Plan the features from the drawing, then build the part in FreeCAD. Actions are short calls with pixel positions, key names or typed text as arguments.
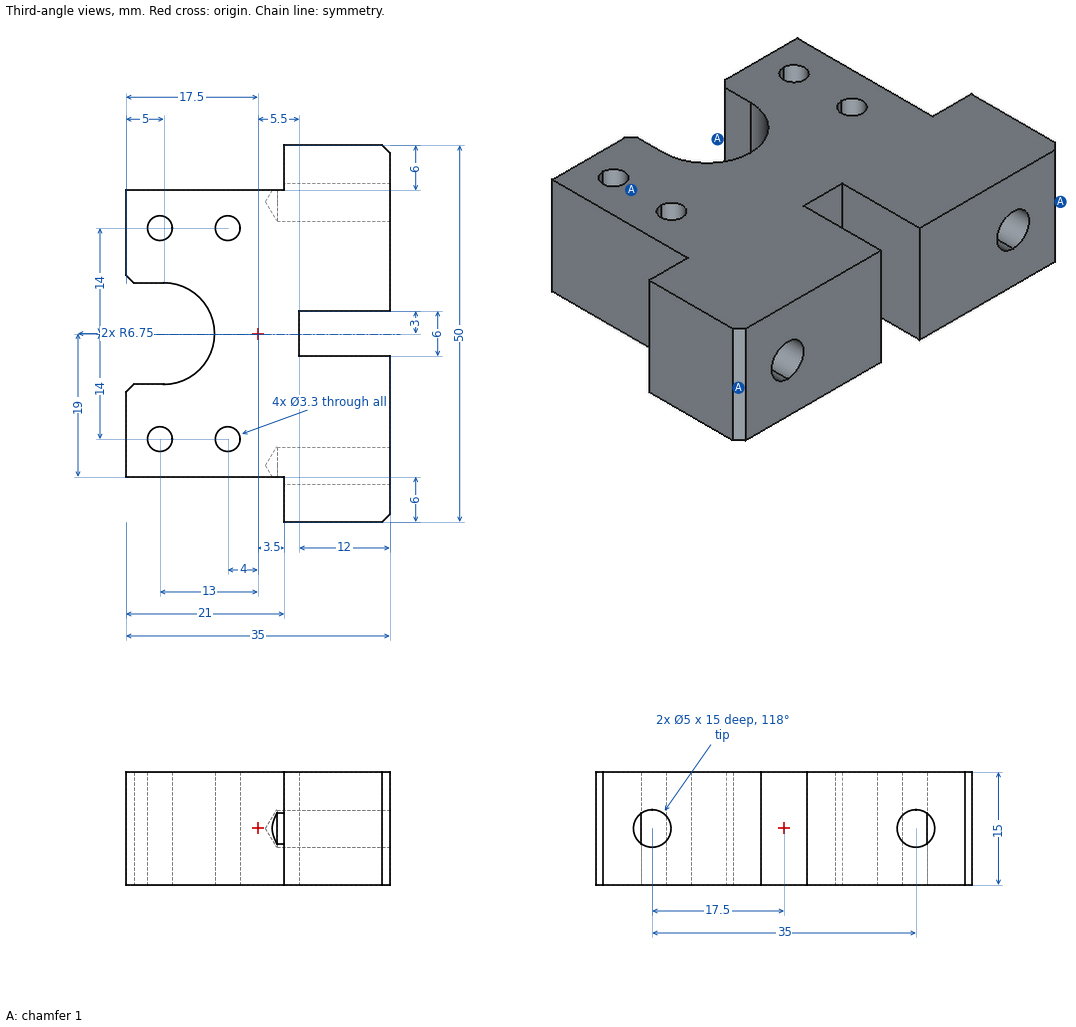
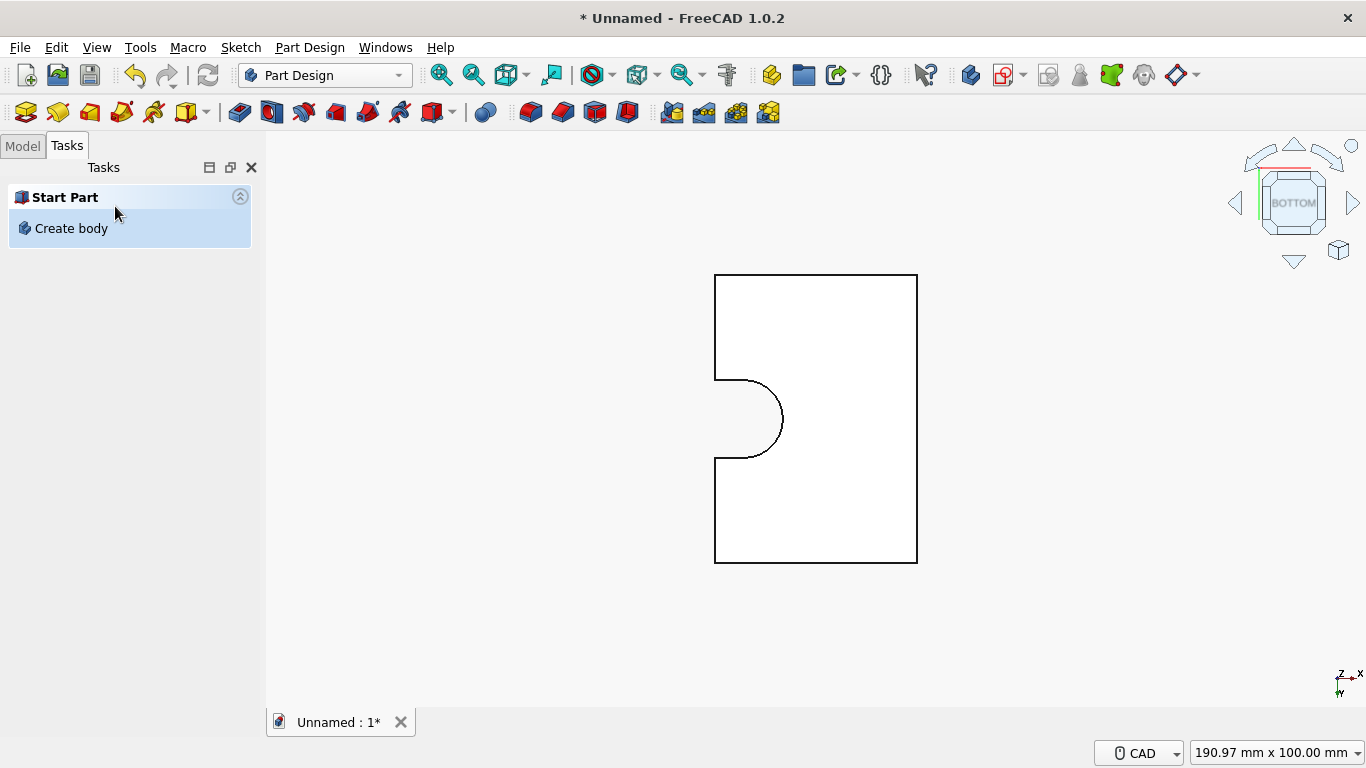
click(845, 459)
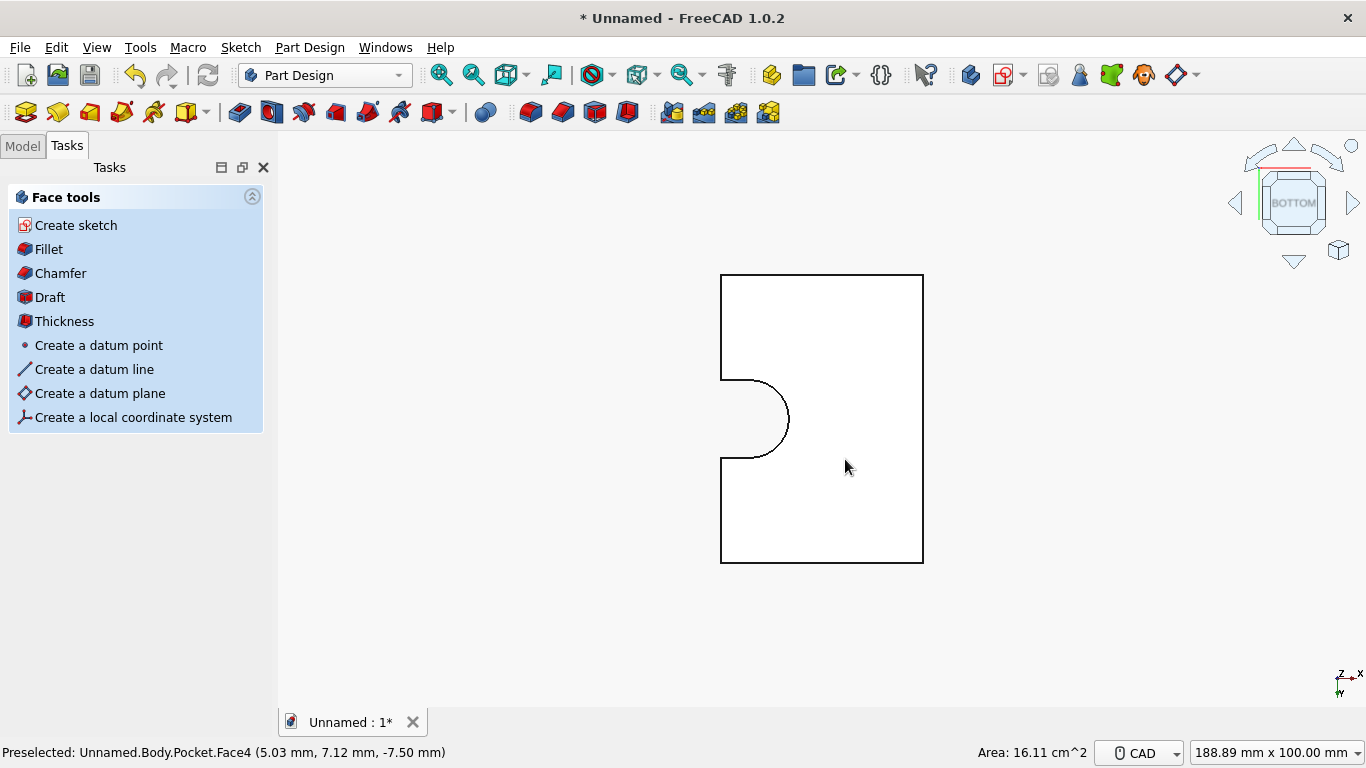
click(1004, 76)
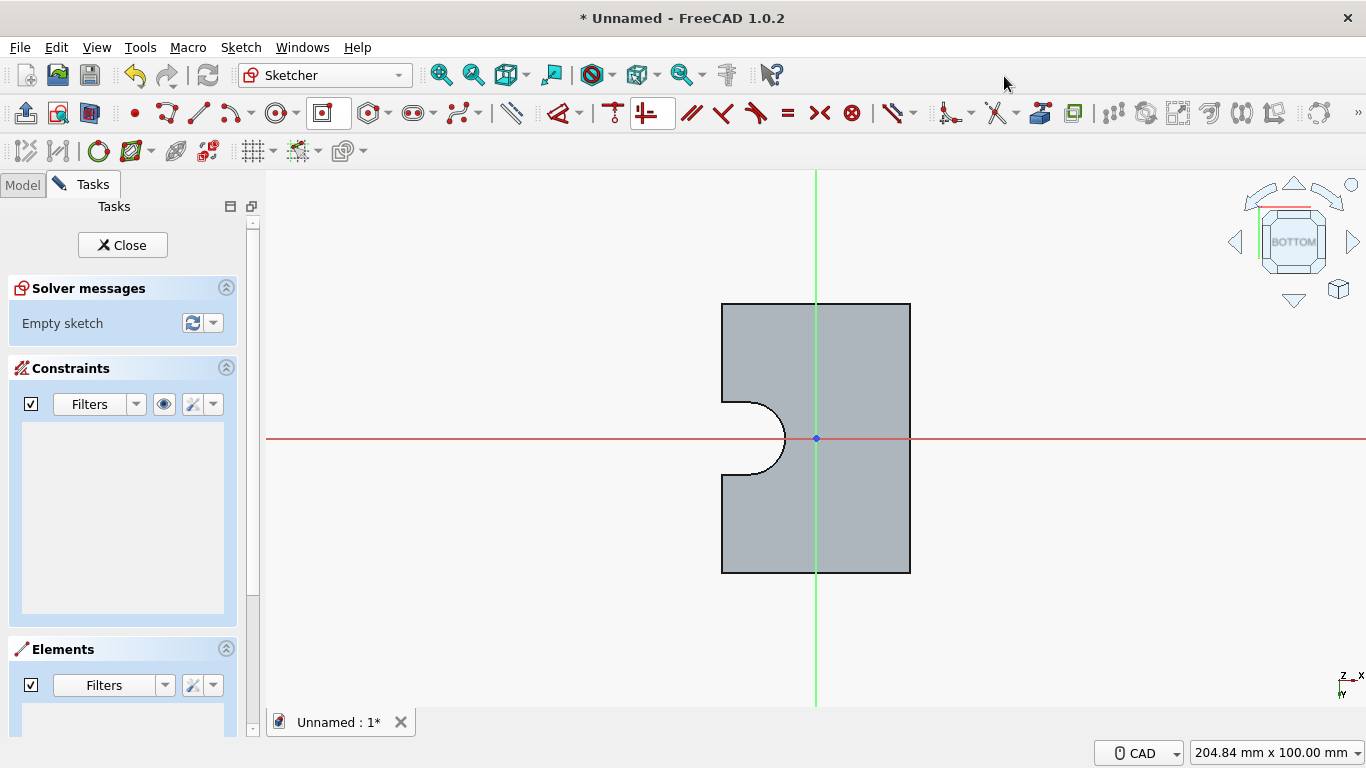
scroll(800, 438, up, 4)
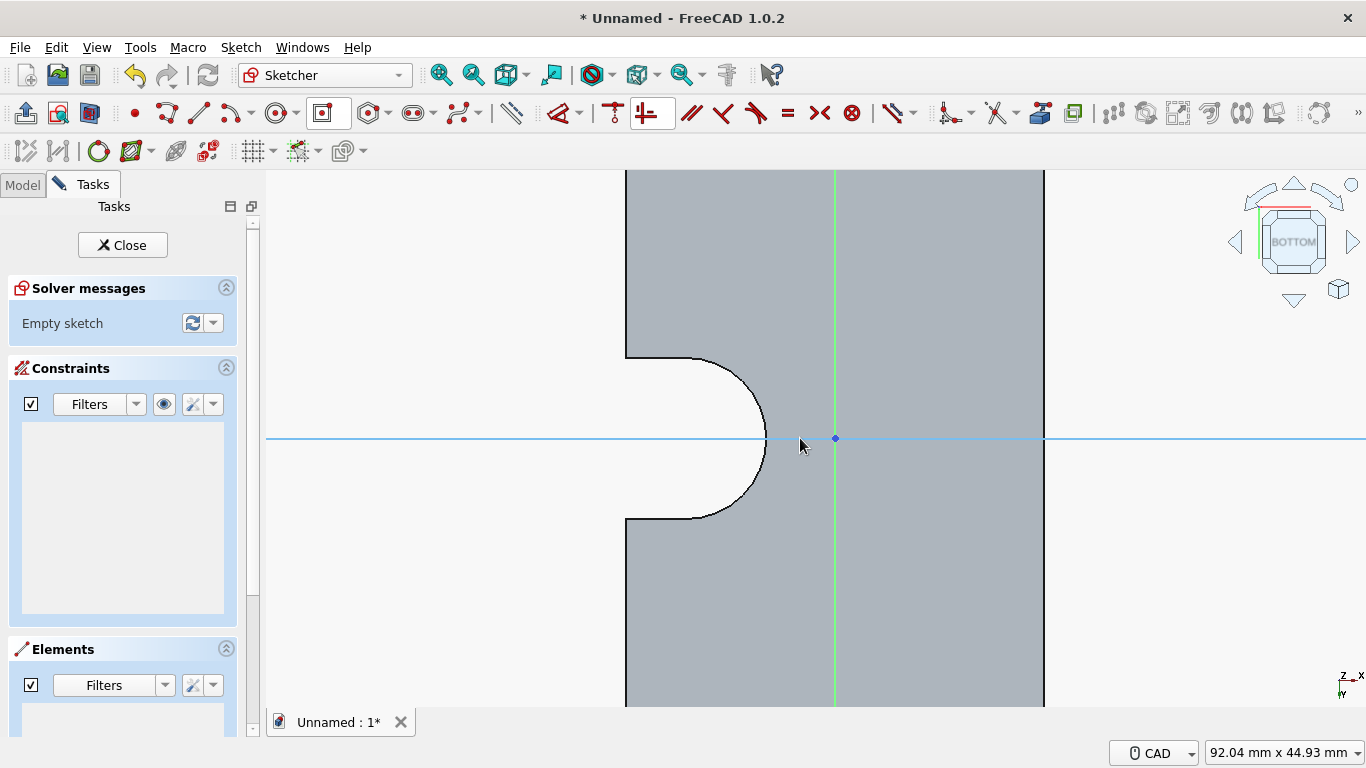
click(276, 114)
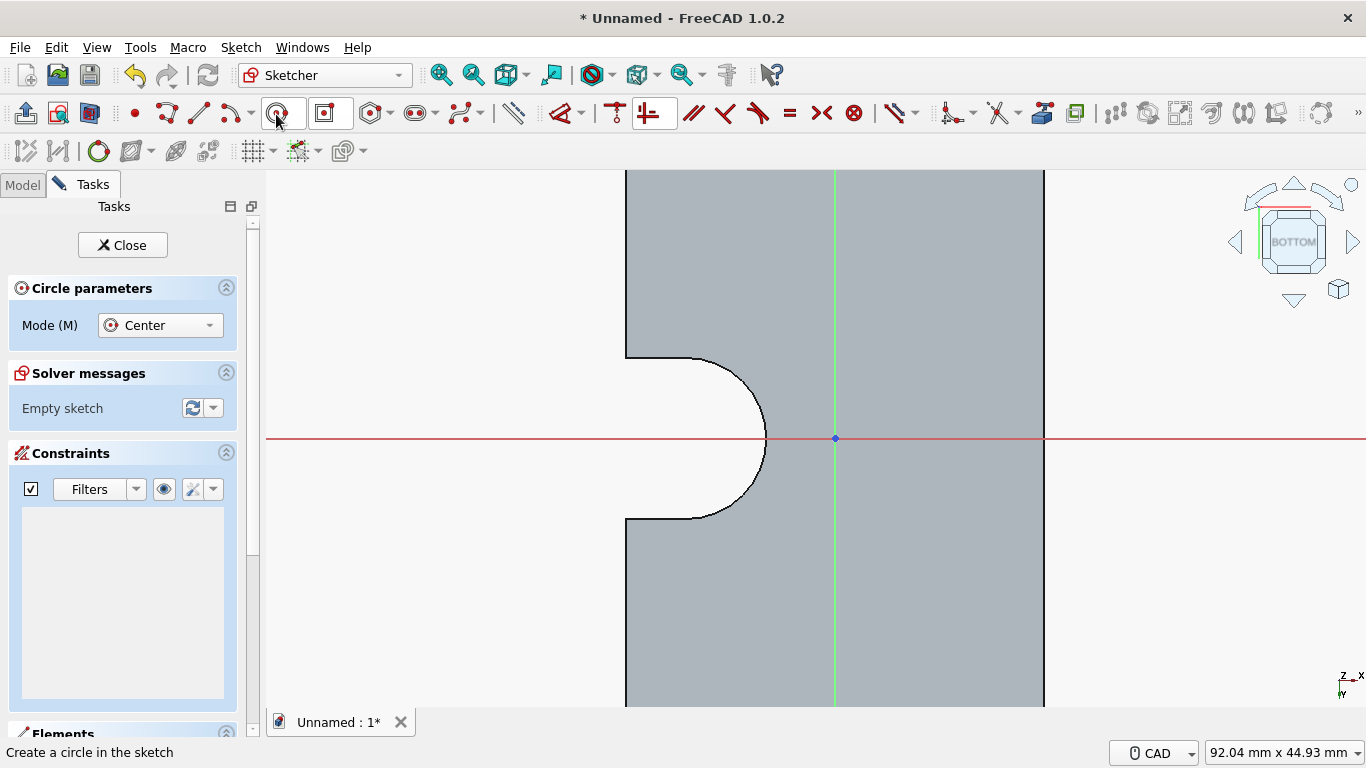
click(787, 271)
move(801, 257)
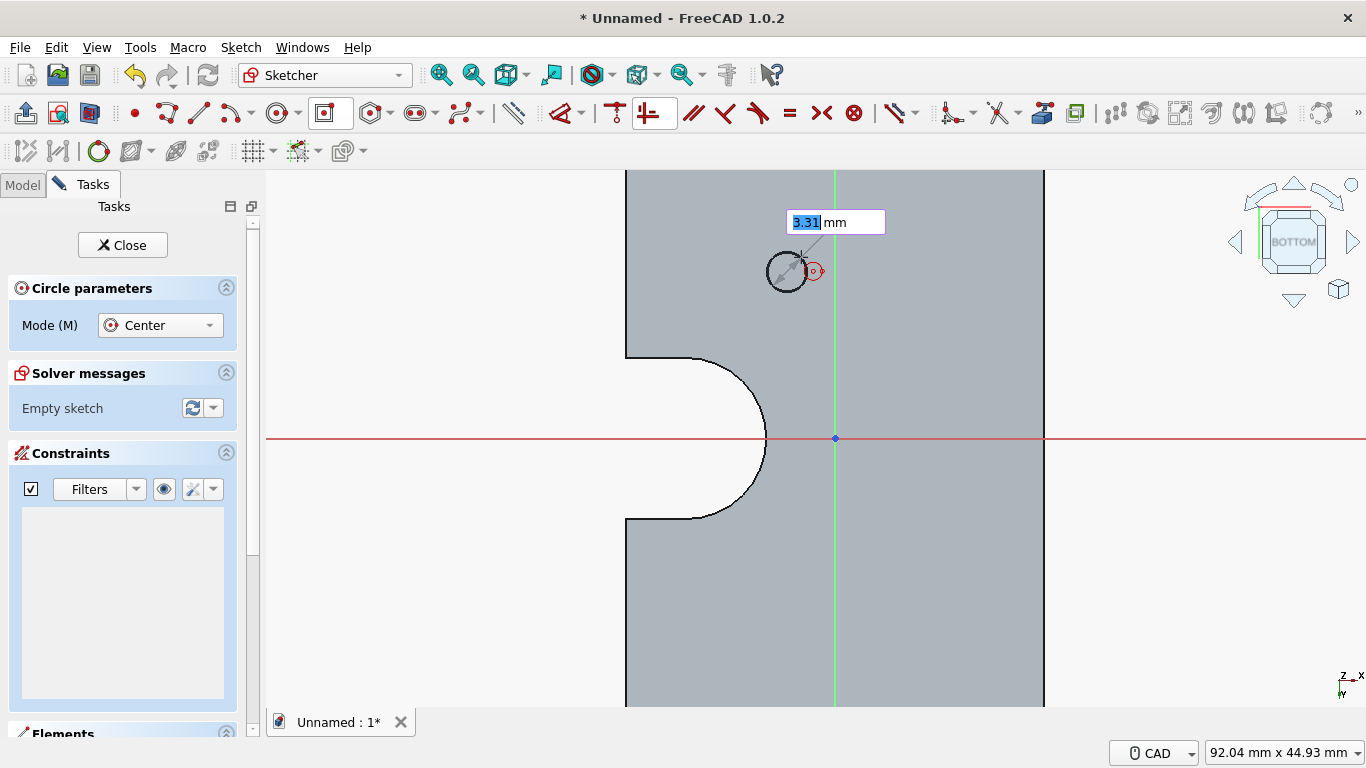
text(3.3)
key(Return)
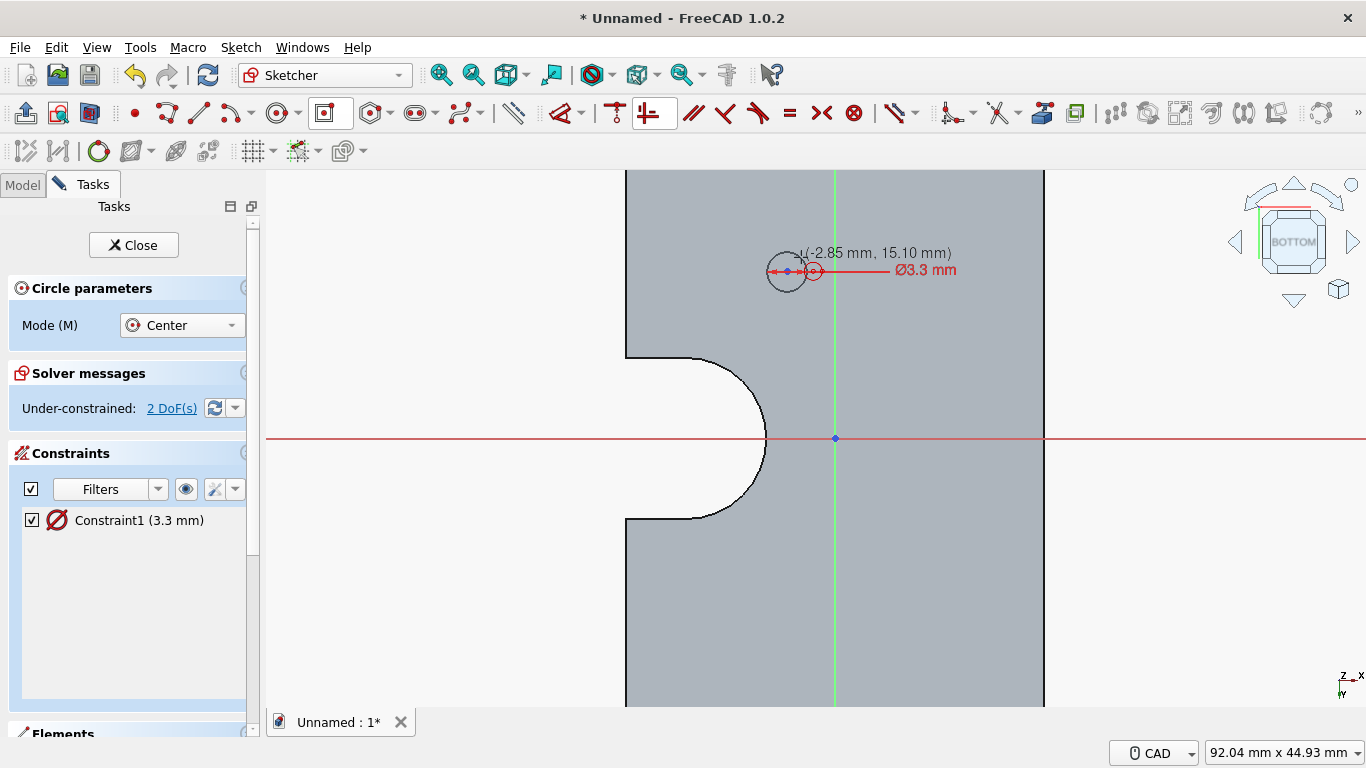
click(680, 271)
move(694, 257)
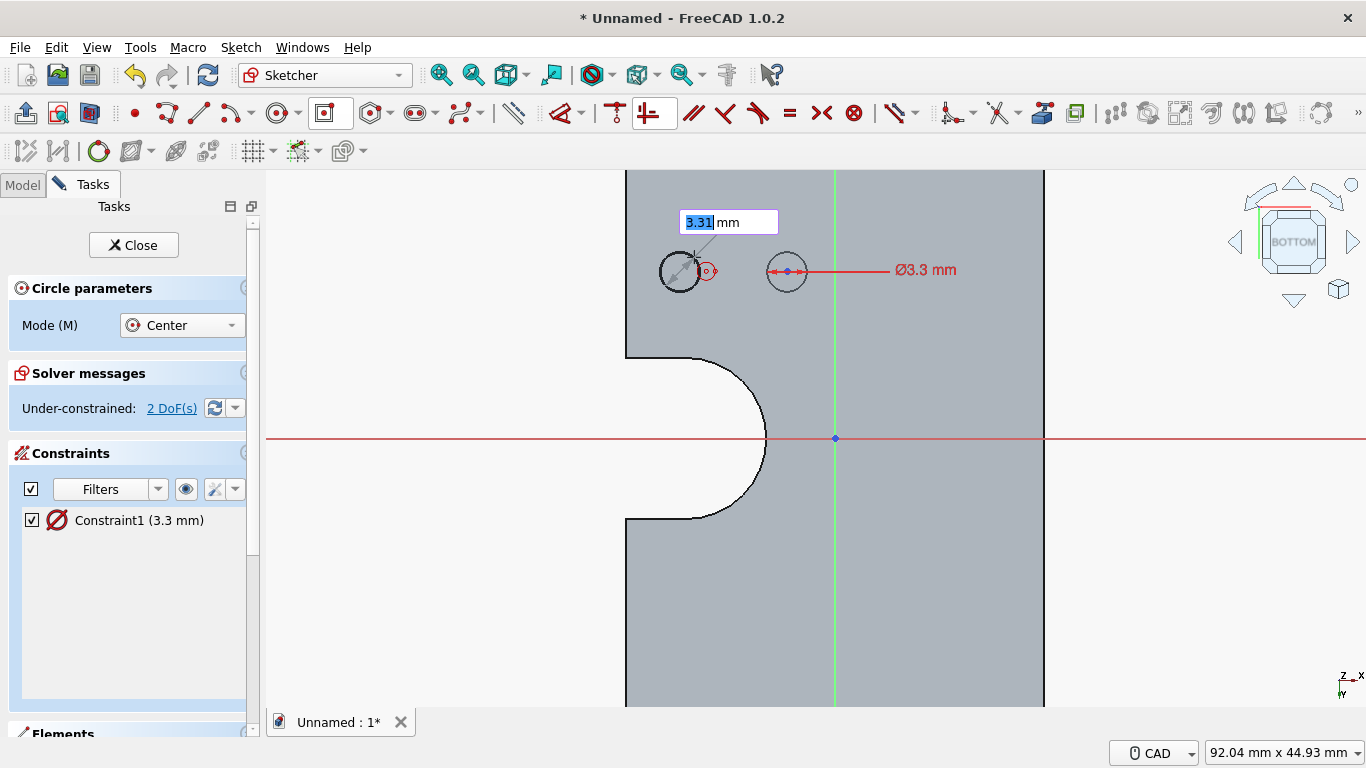
text(3.3)
key(Return)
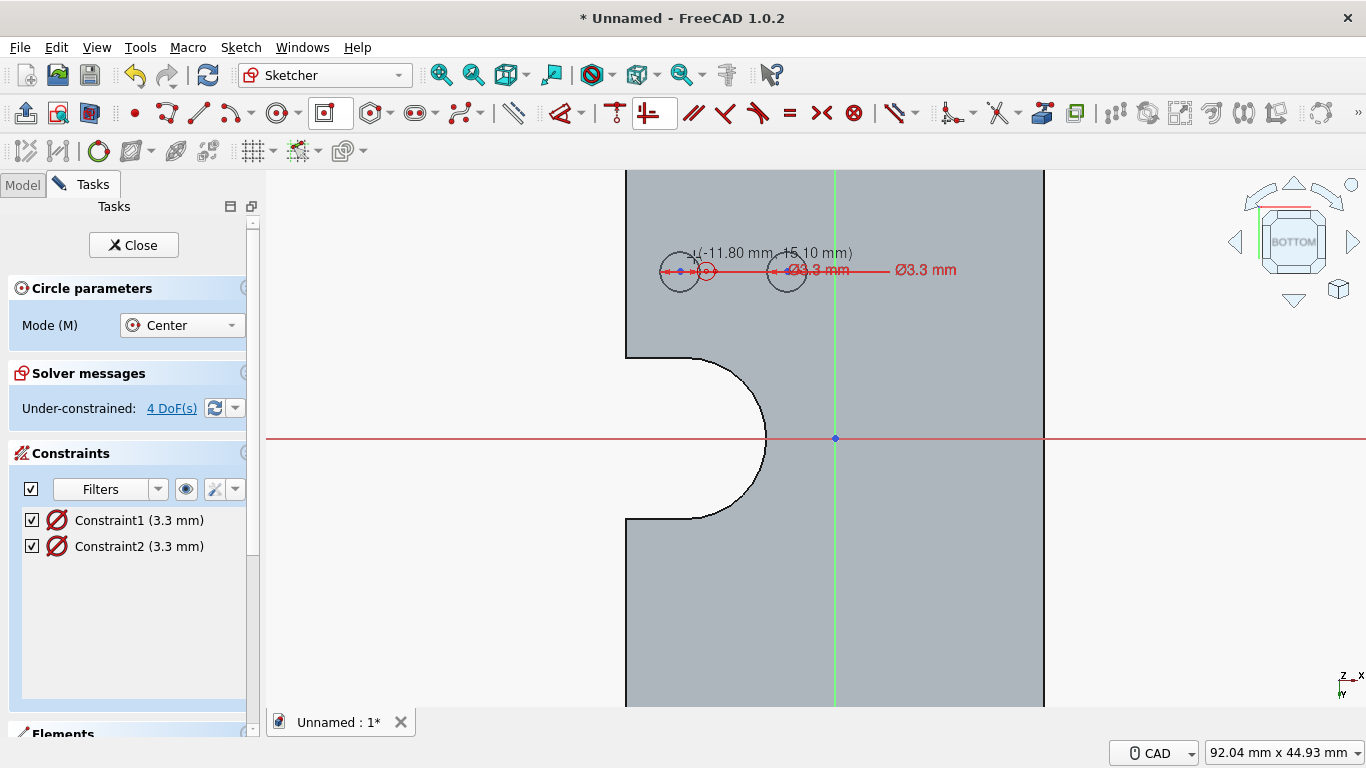
click(787, 606)
move(801, 592)